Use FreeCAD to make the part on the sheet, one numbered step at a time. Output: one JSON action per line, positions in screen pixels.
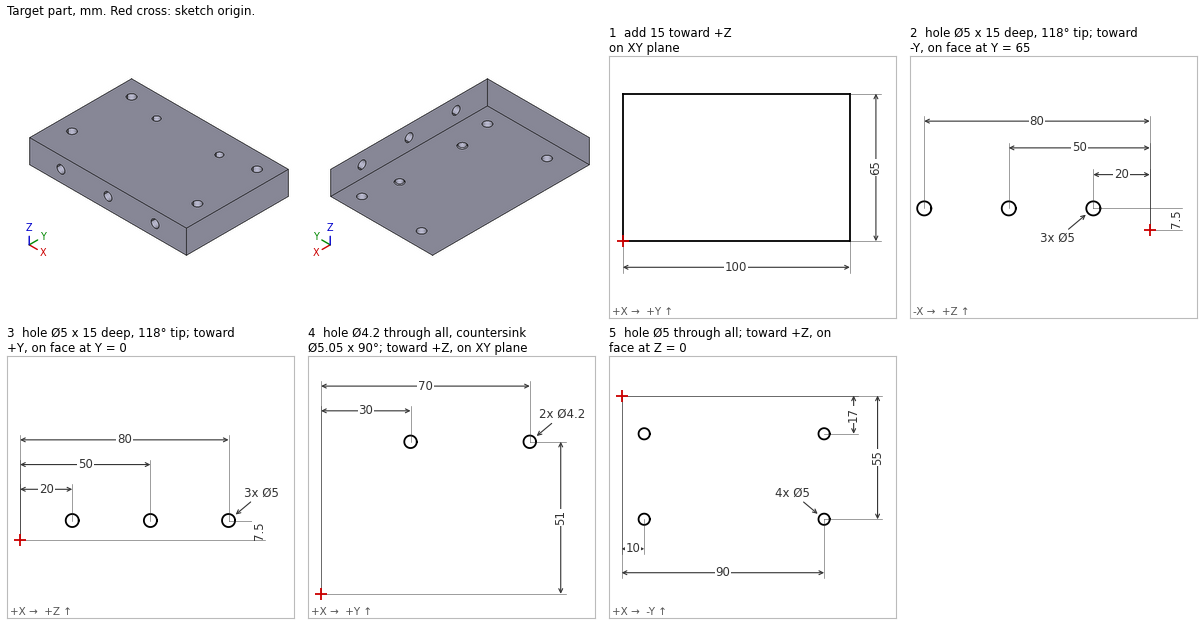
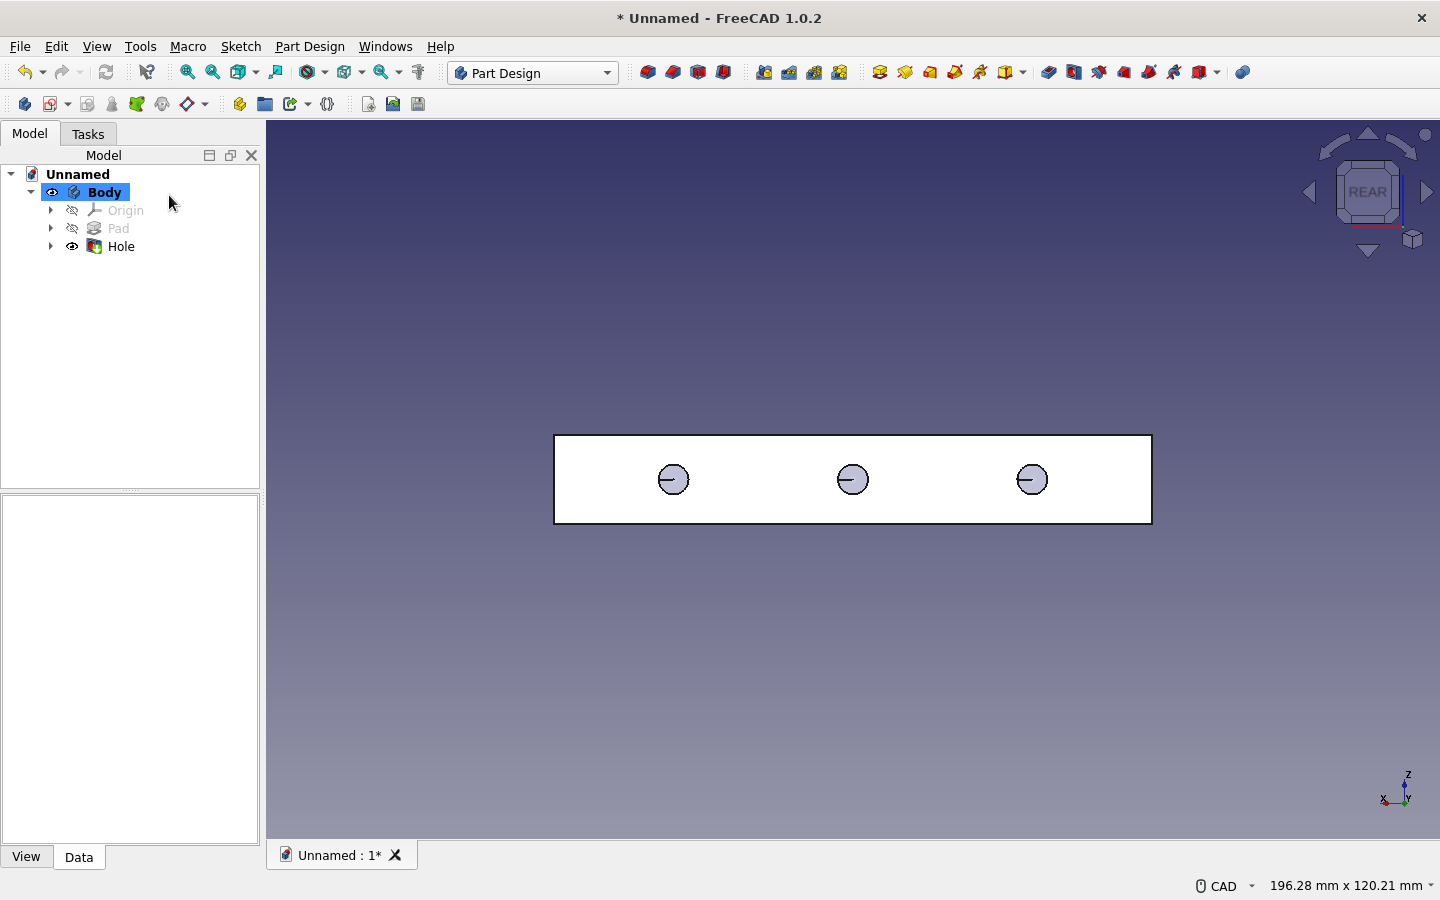
{"action": "key", "text": "0"}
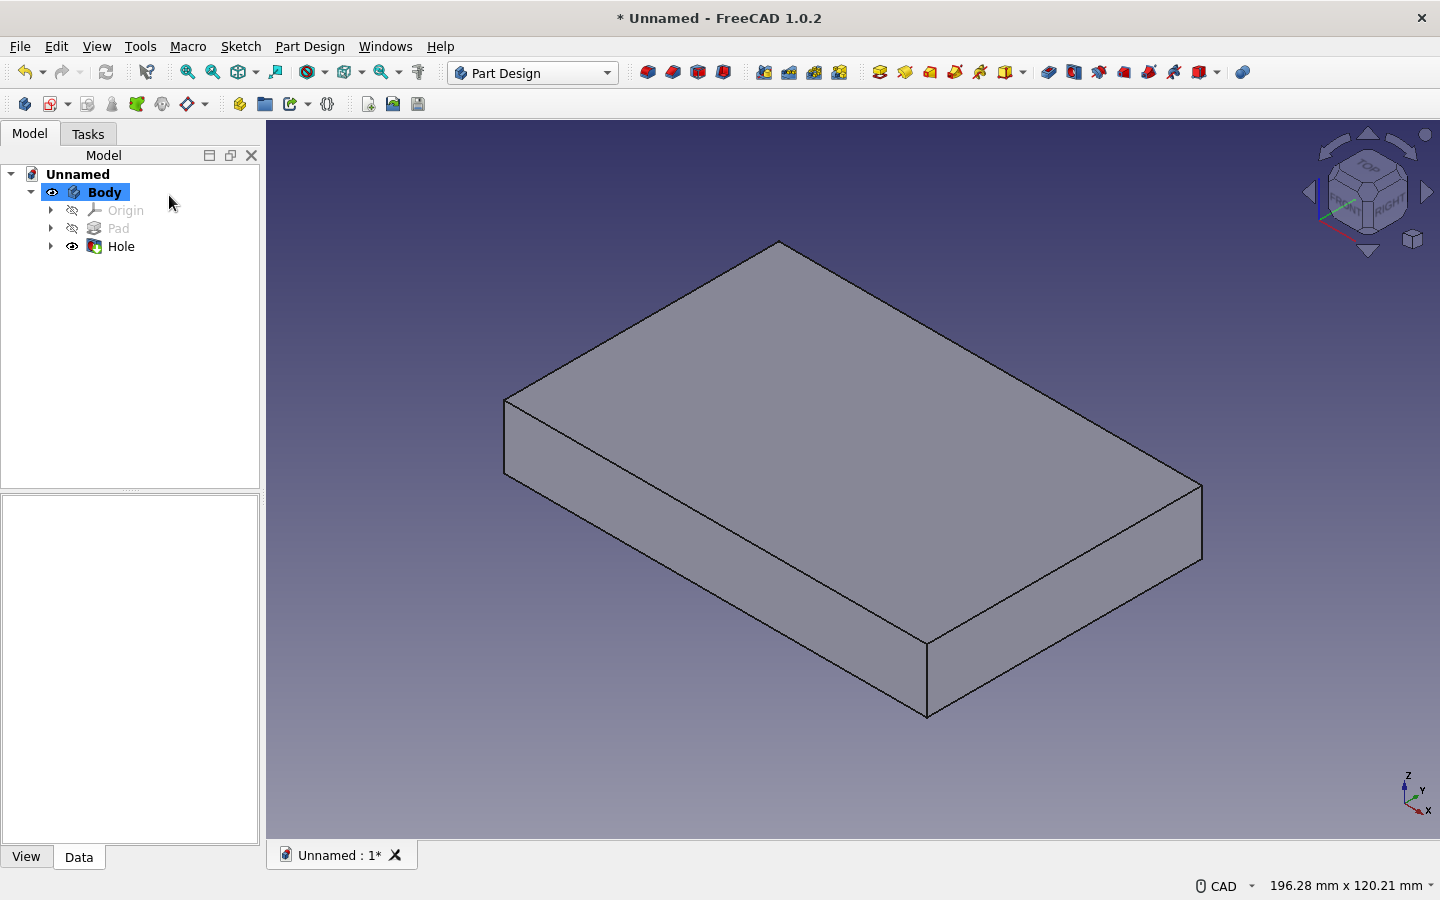
{"action": "left_click", "coordinate": [836, 628]}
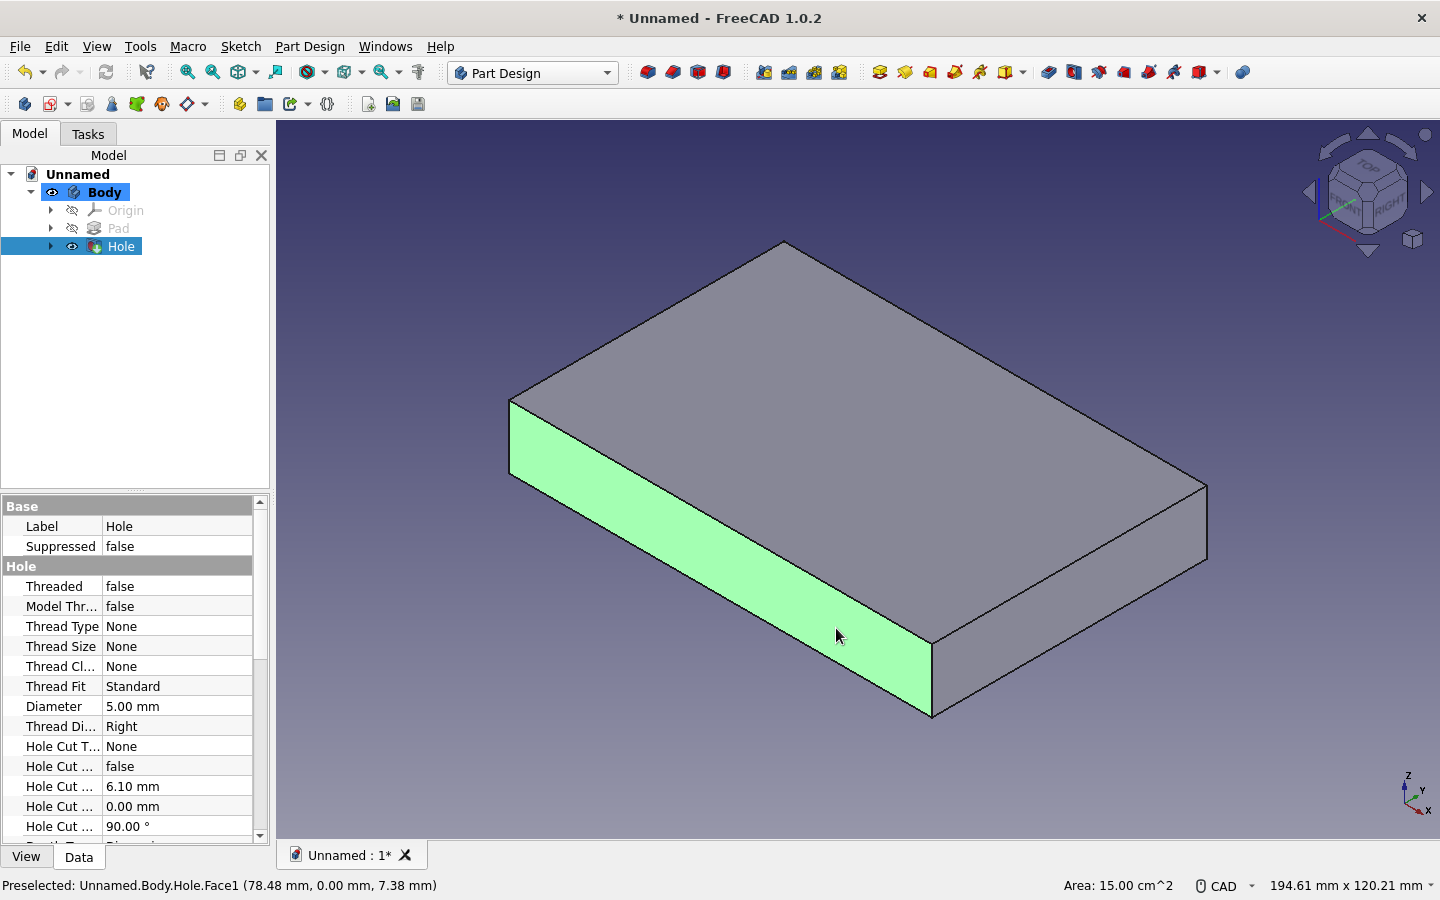
{"action": "left_click", "coordinate": [50, 104]}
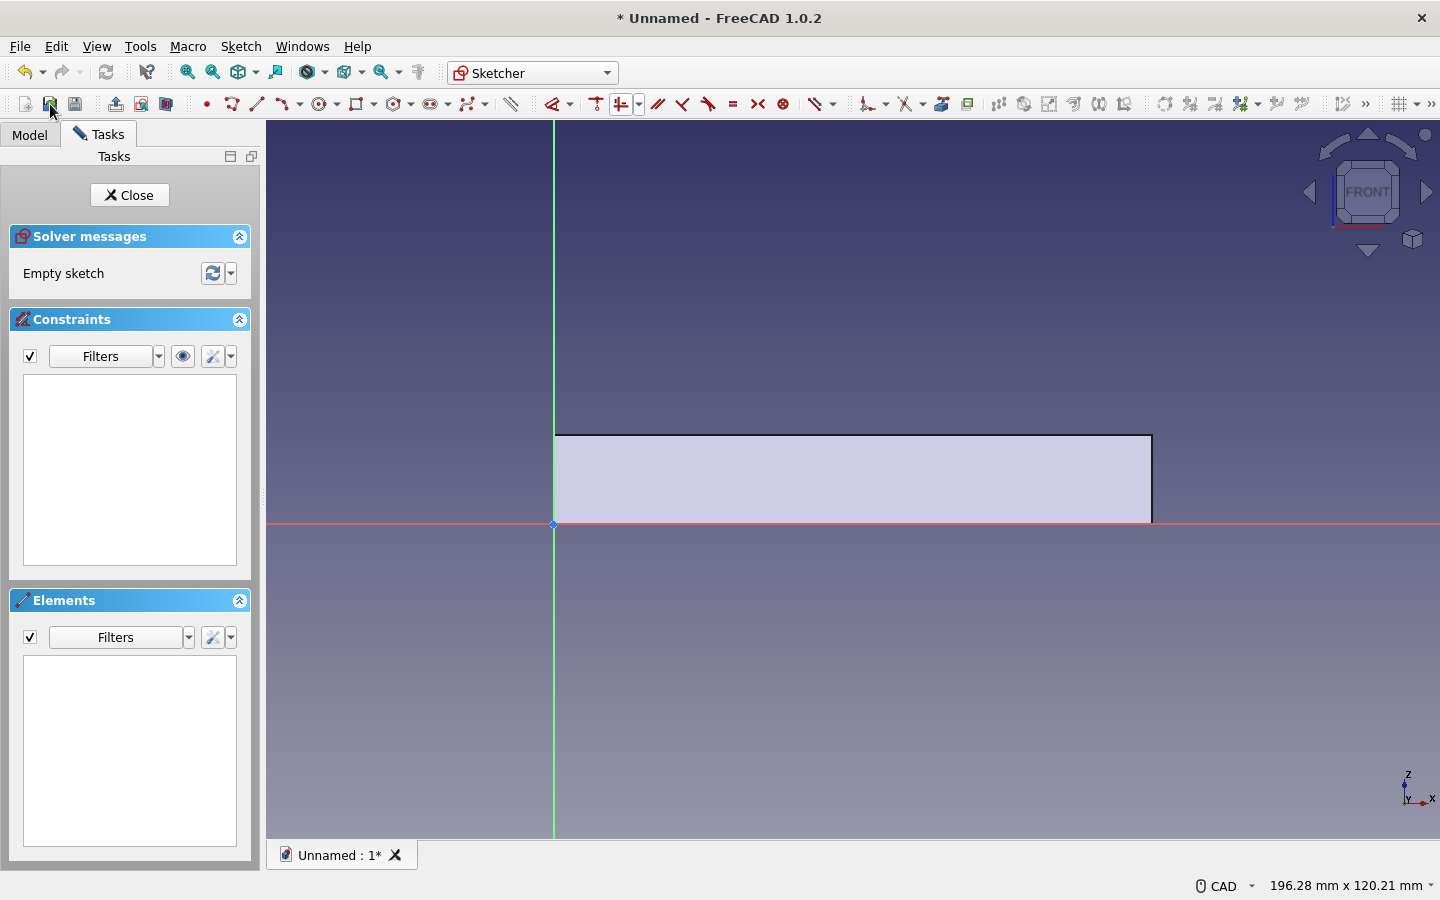
{"action": "scroll", "coordinate": [834, 525], "scroll_direction": "up", "scroll_amount": 2}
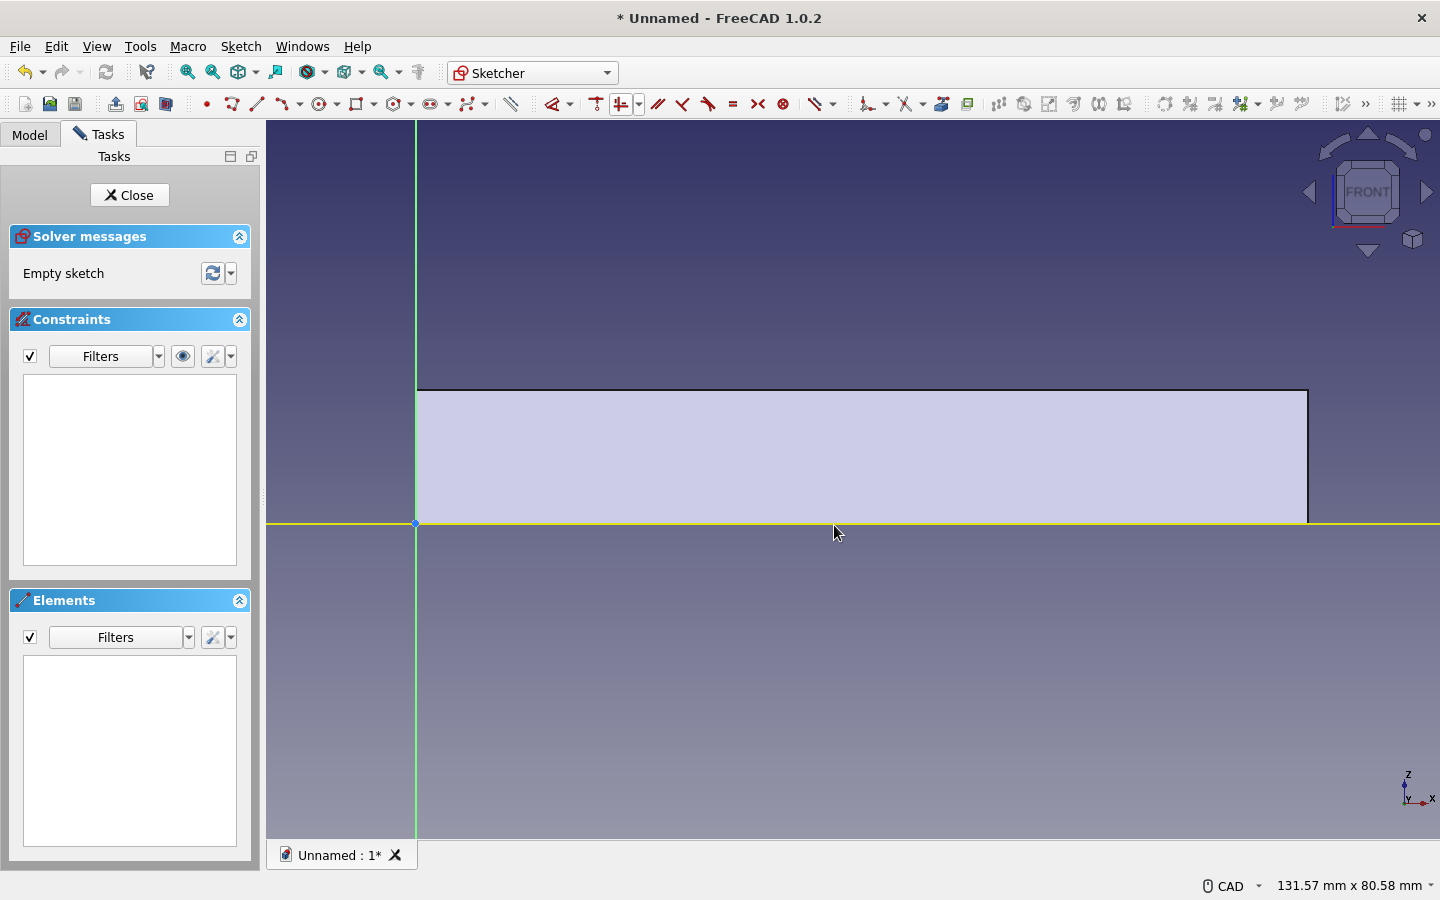
{"action": "left_click", "coordinate": [318, 104]}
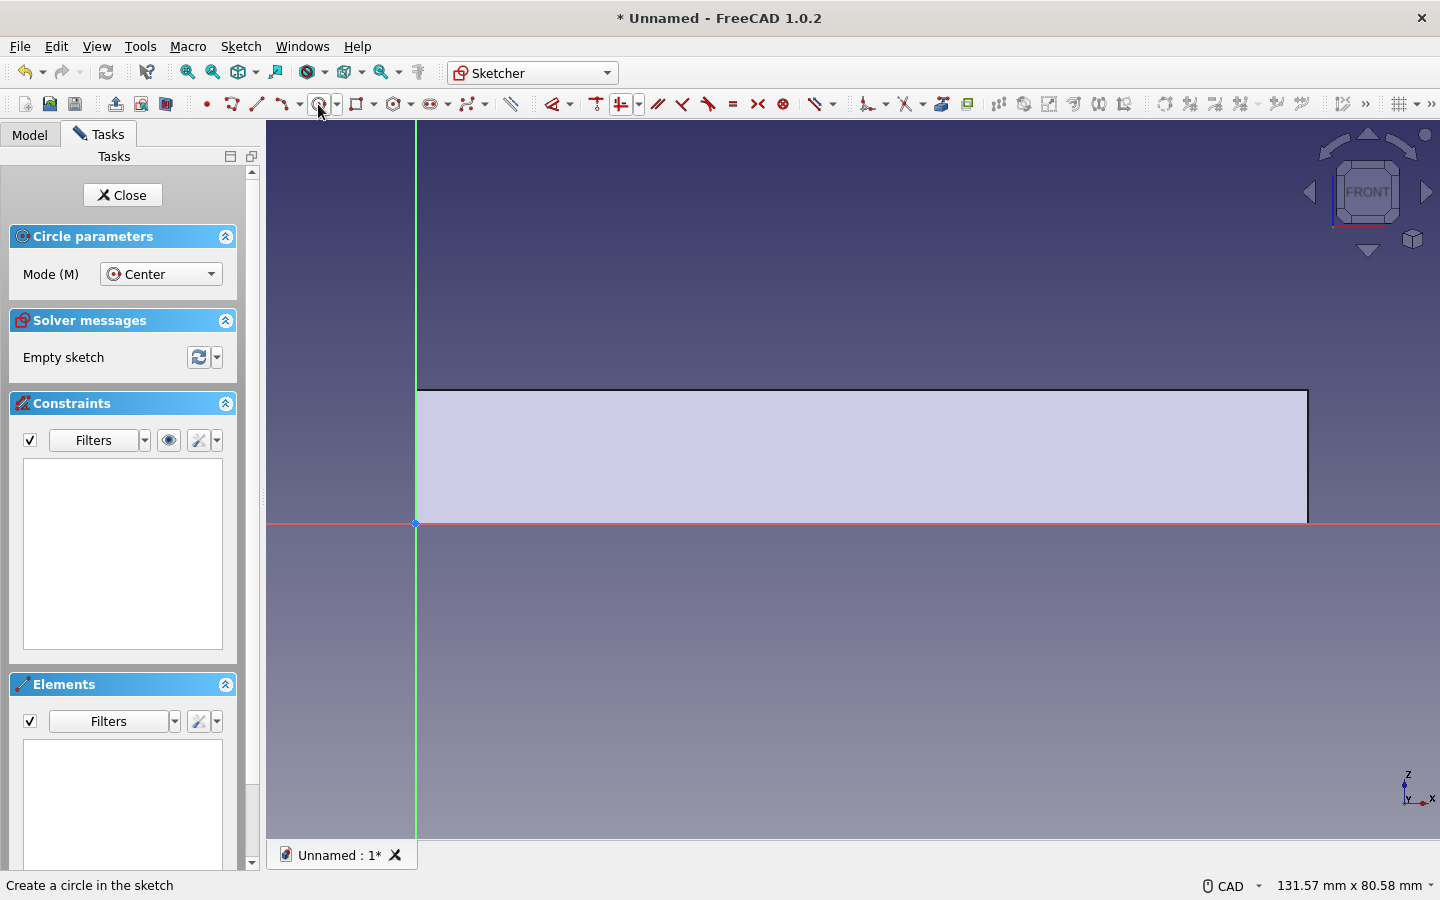
{"action": "left_click", "coordinate": [1130, 457]}
{"action": "mouse_move", "coordinate": [1146, 441]}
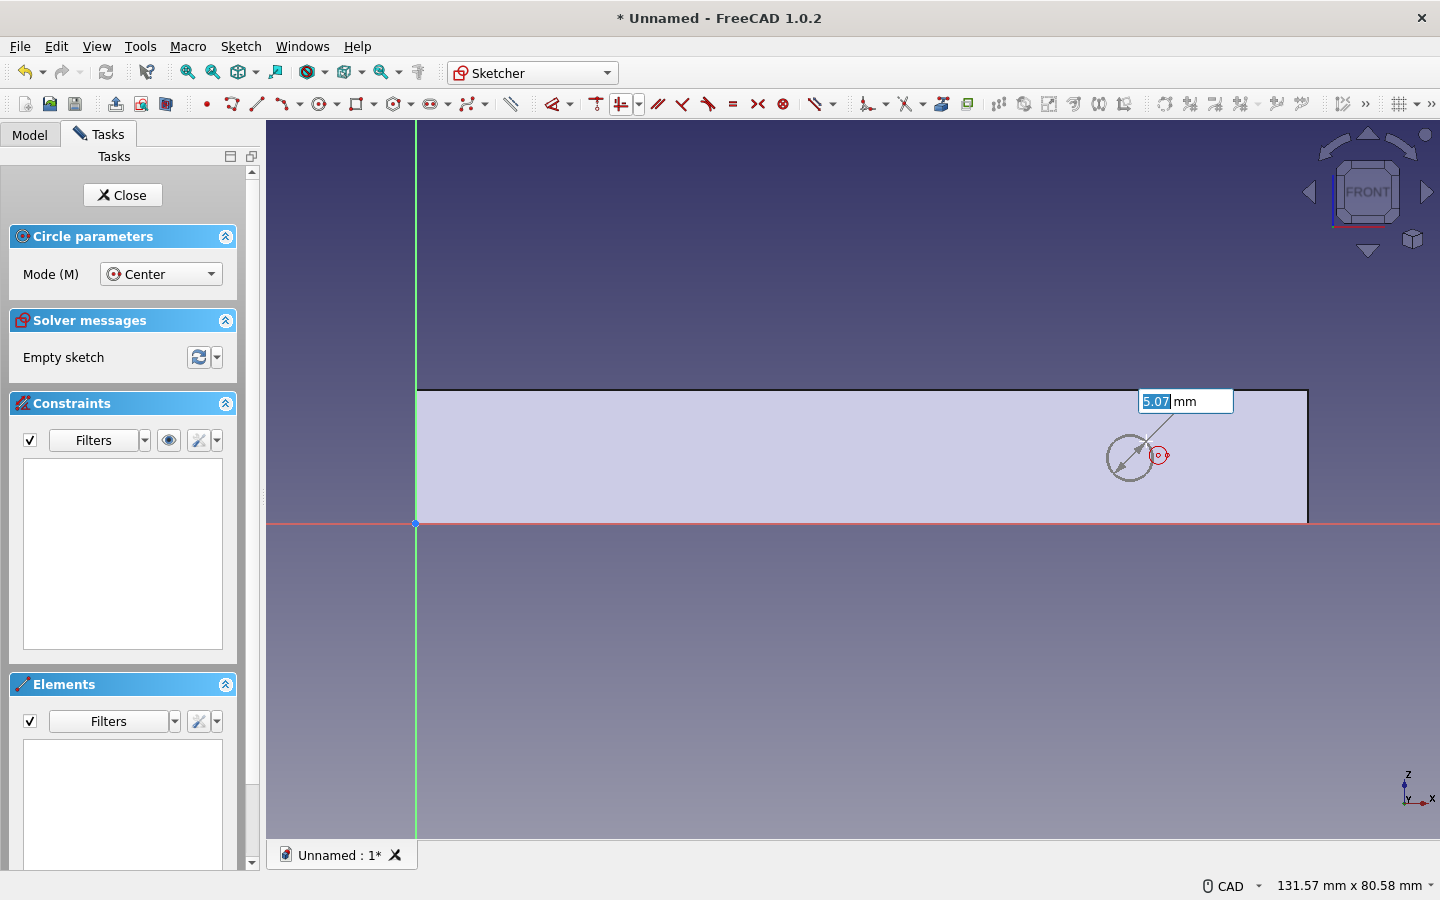
{"action": "type", "text": "5"}
{"action": "key", "text": "Return"}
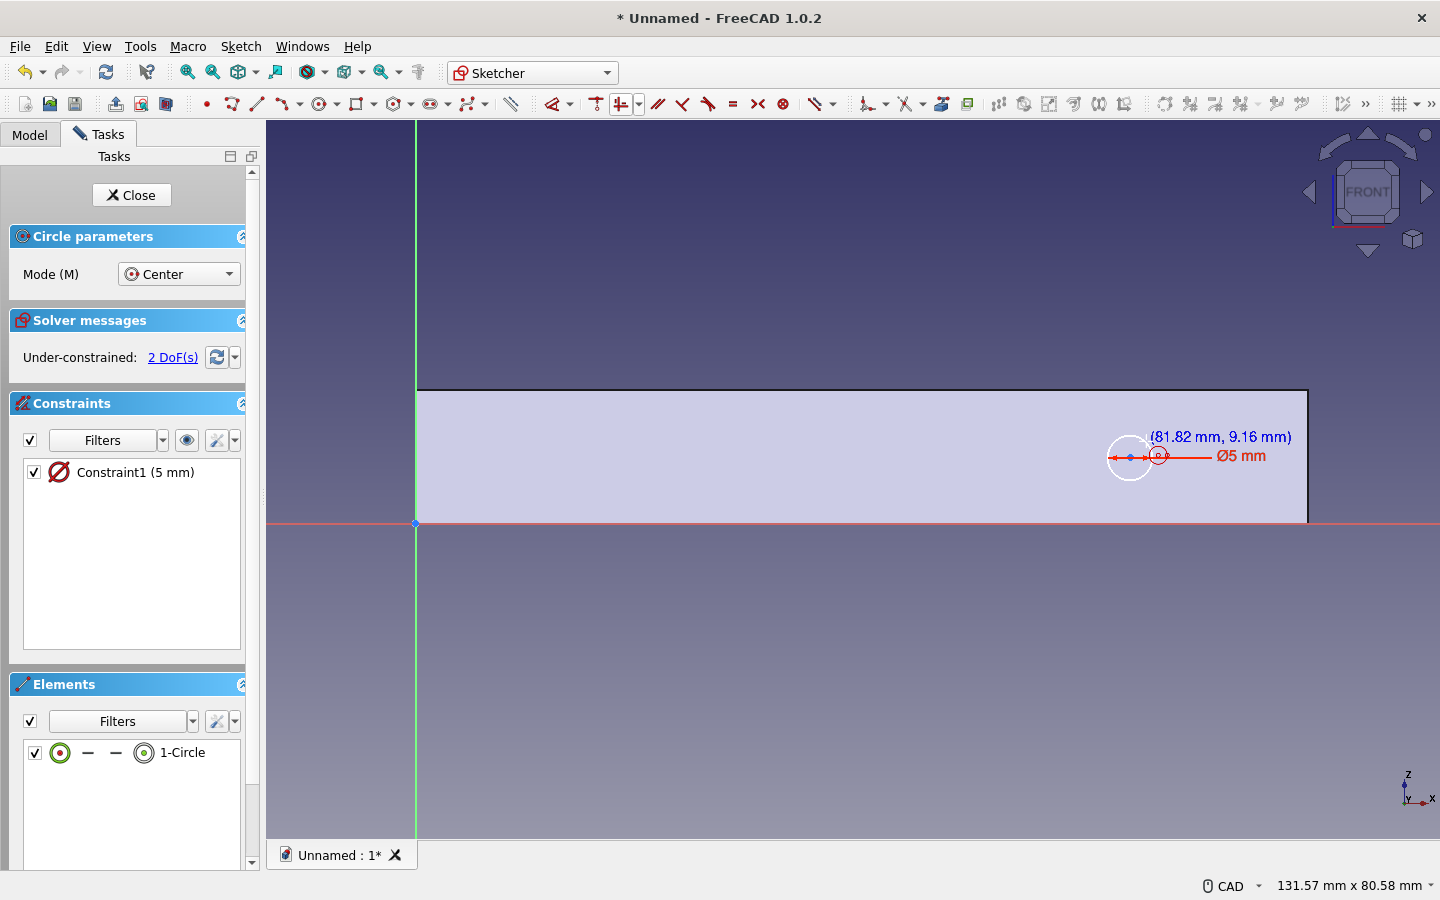
{"action": "left_click", "coordinate": [862, 457]}
{"action": "mouse_move", "coordinate": [878, 441]}